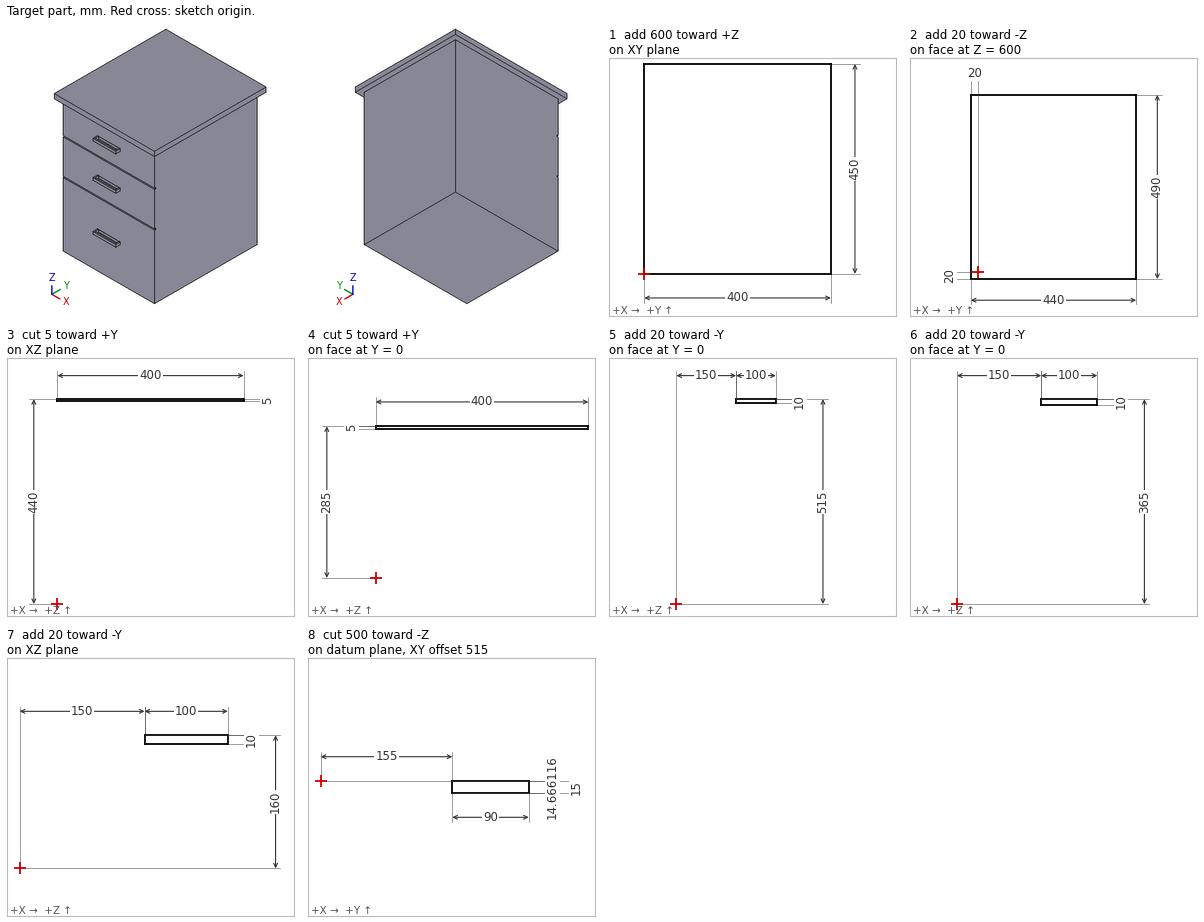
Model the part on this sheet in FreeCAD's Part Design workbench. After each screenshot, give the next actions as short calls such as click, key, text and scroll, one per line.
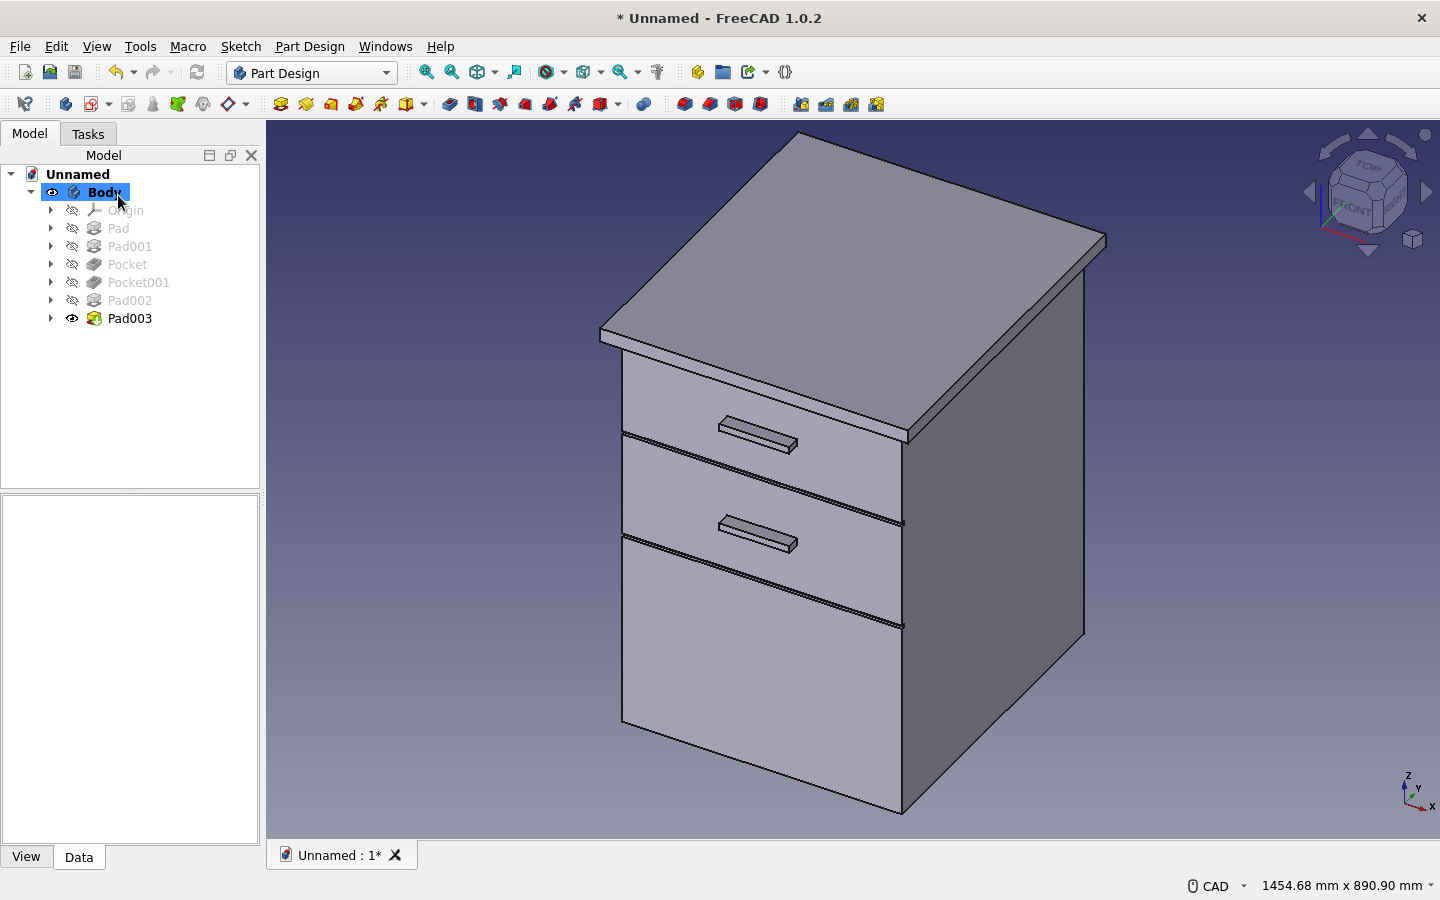
click(90, 104)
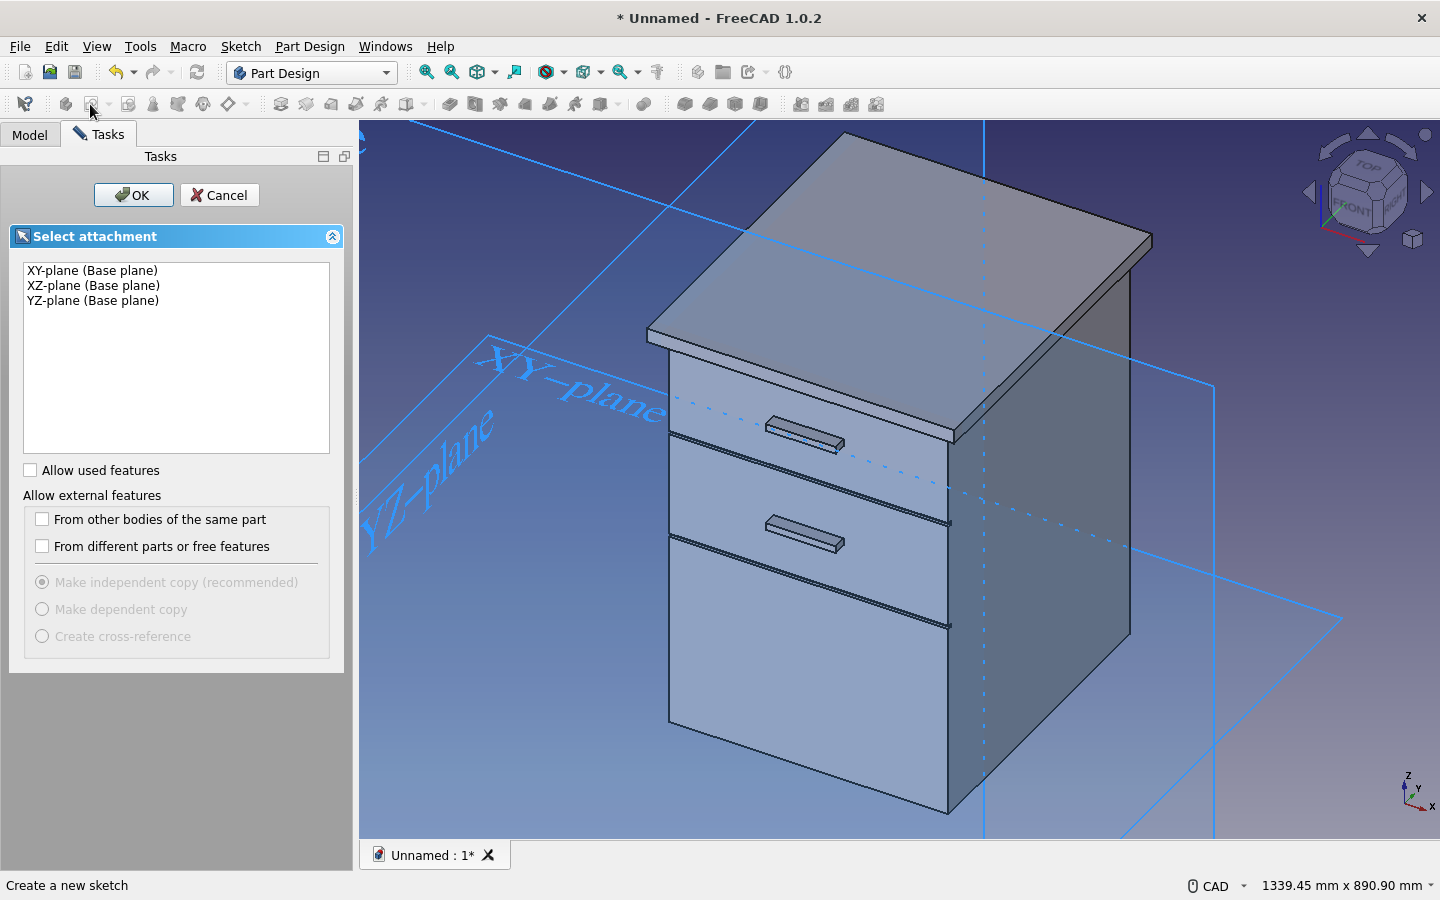
click(84, 286)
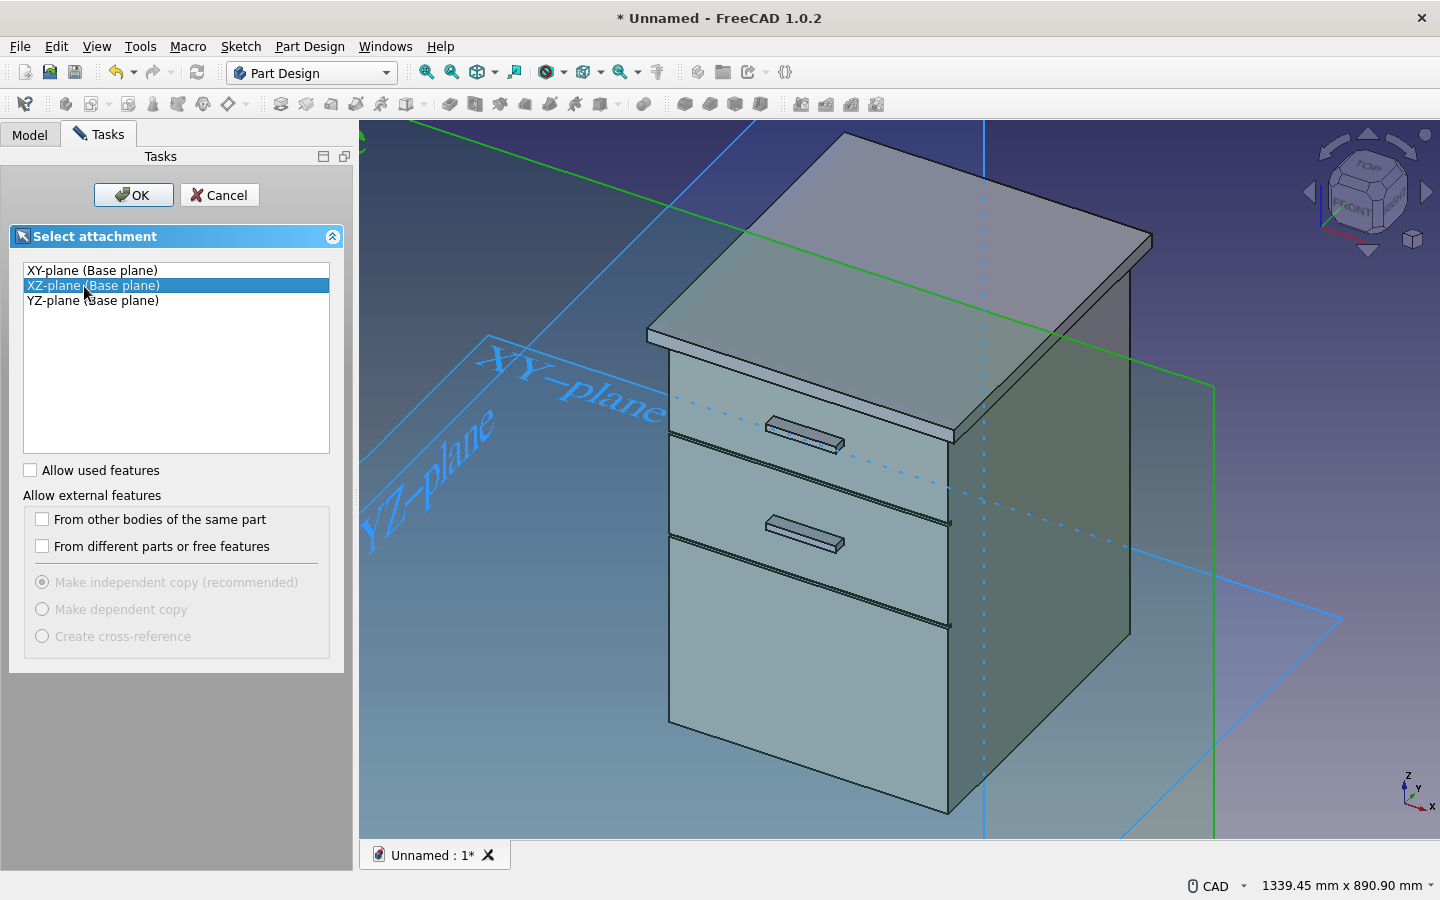
click(134, 195)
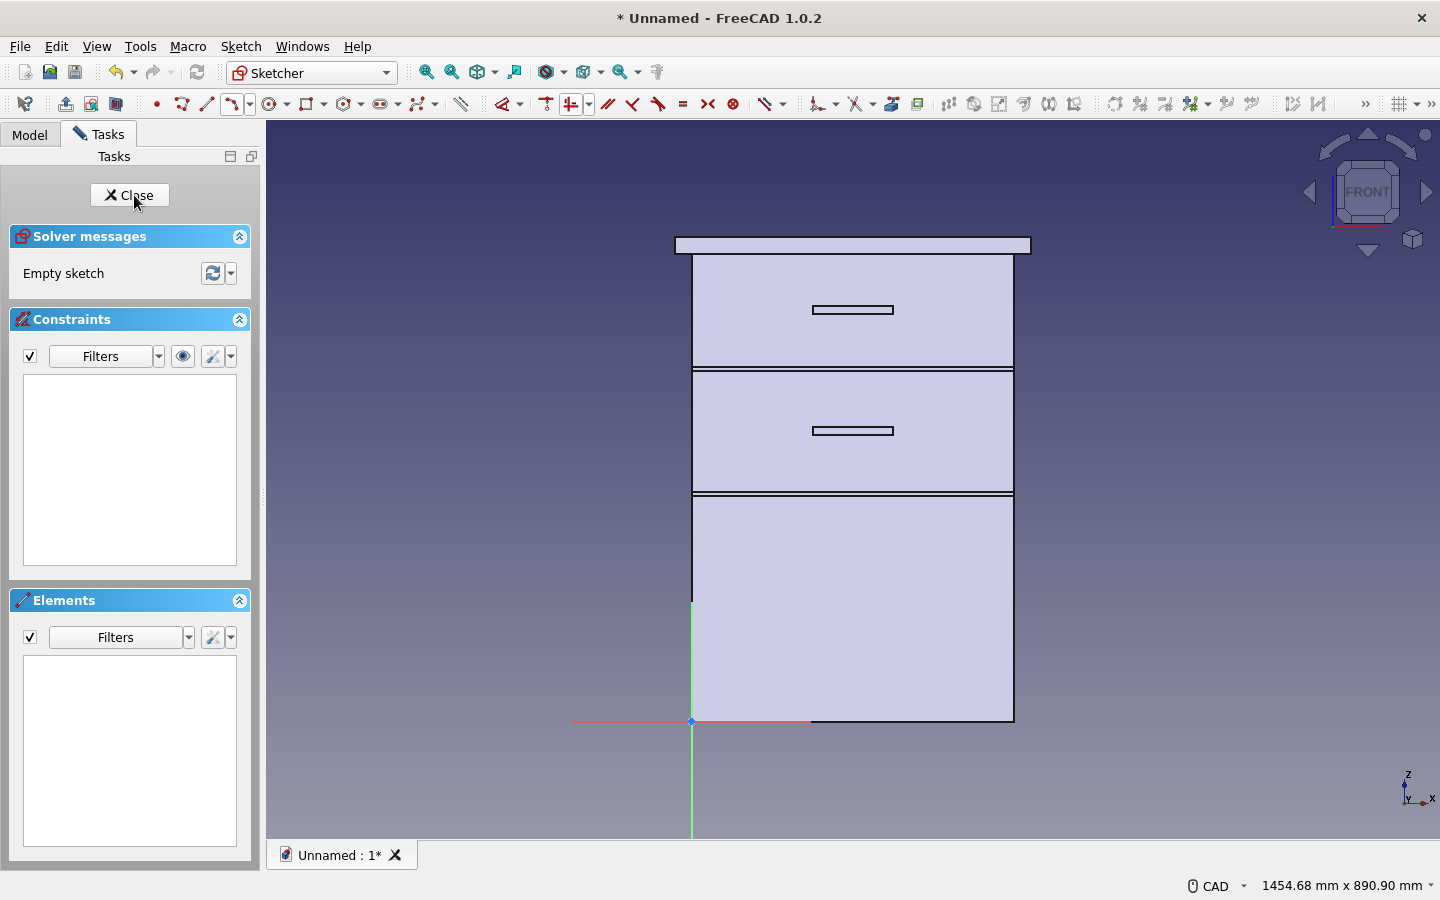
click(116, 104)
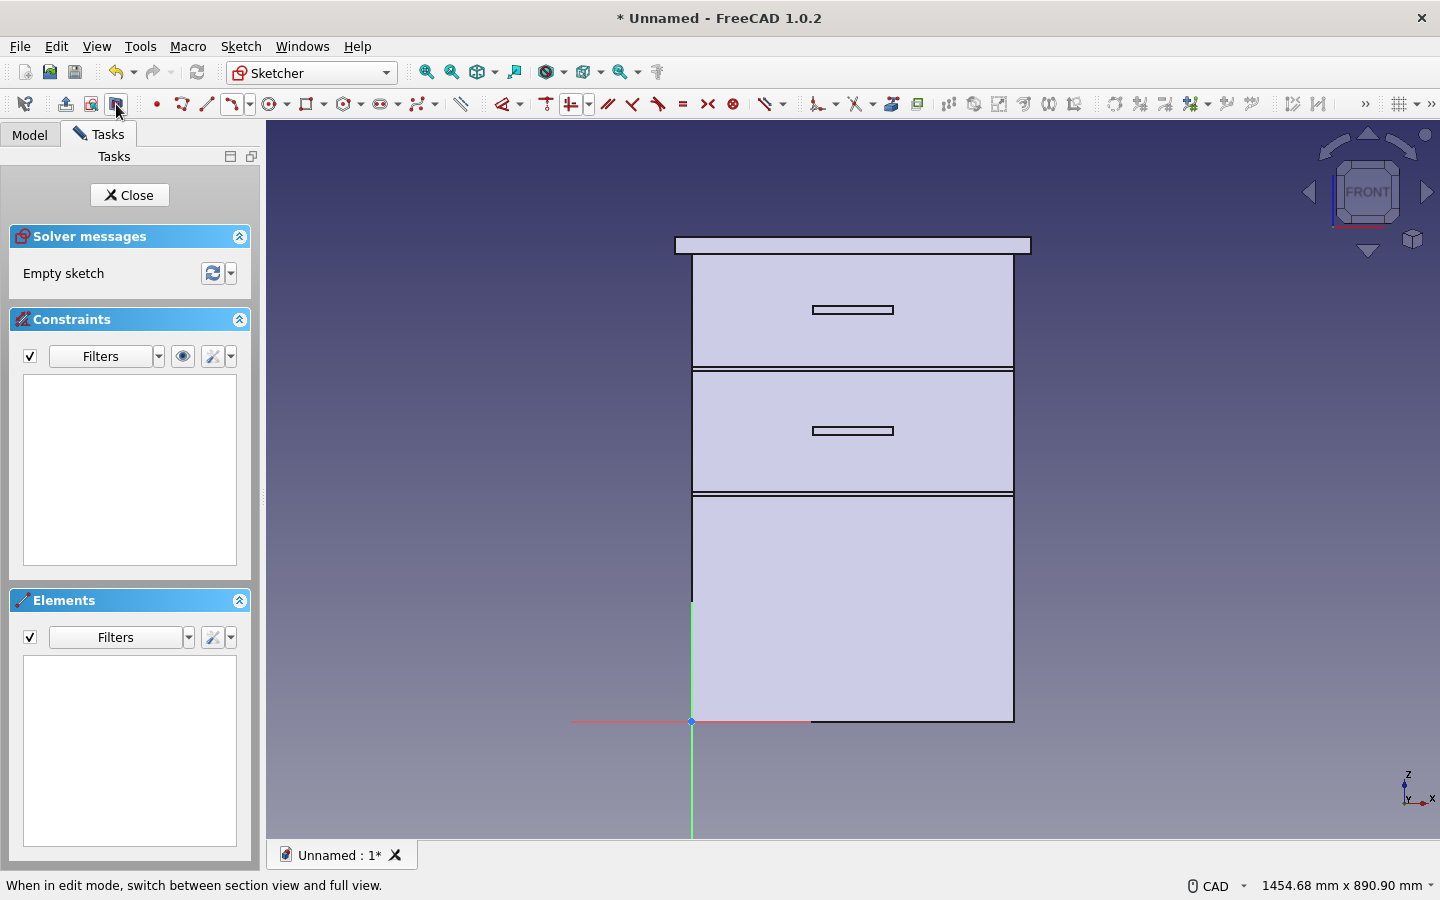
scroll(862, 611, up, 11)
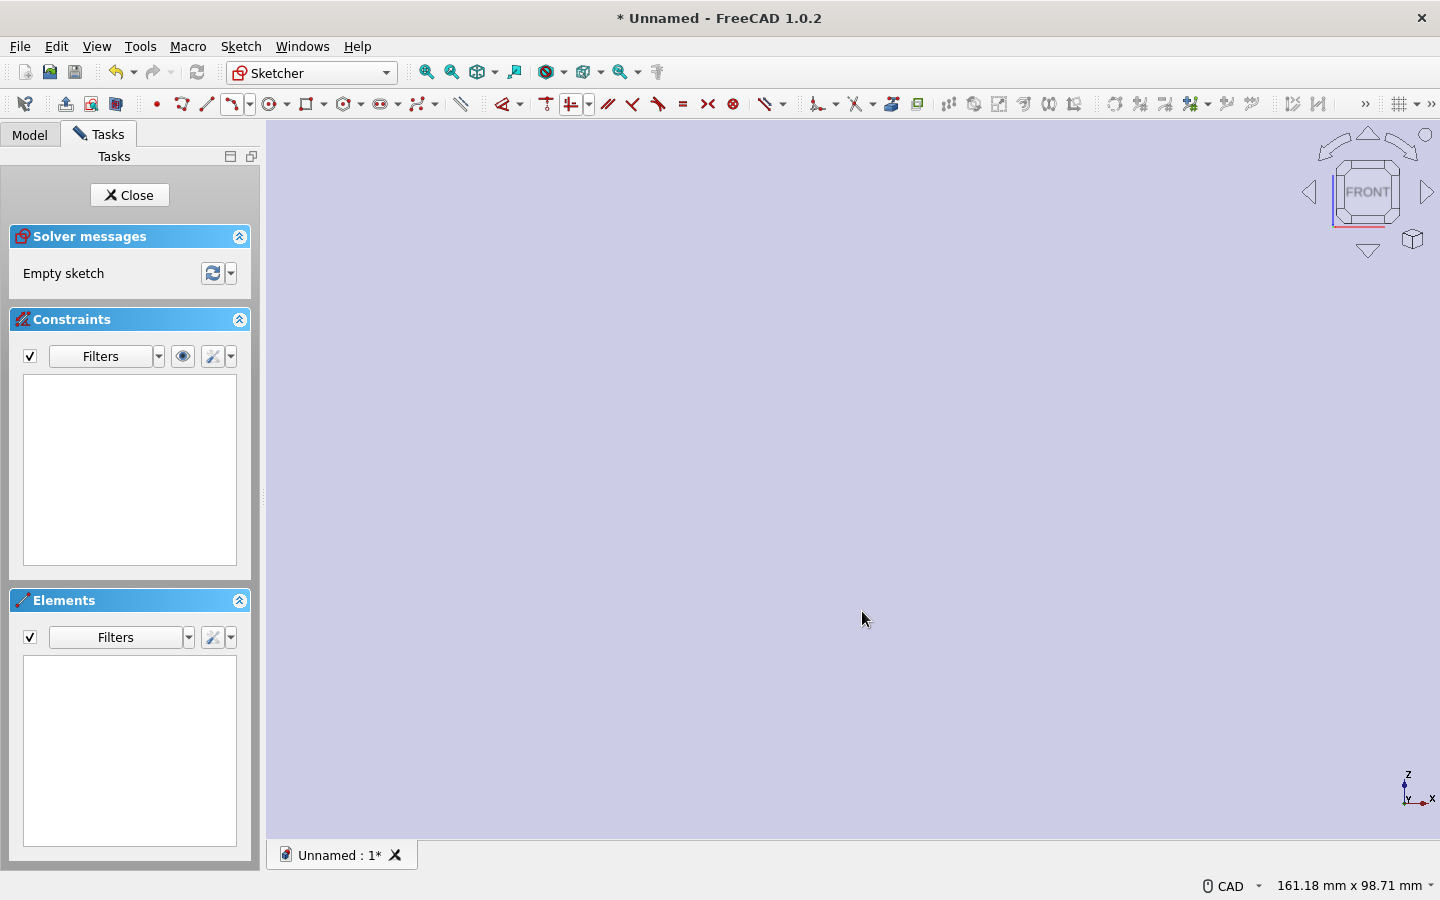
click(306, 104)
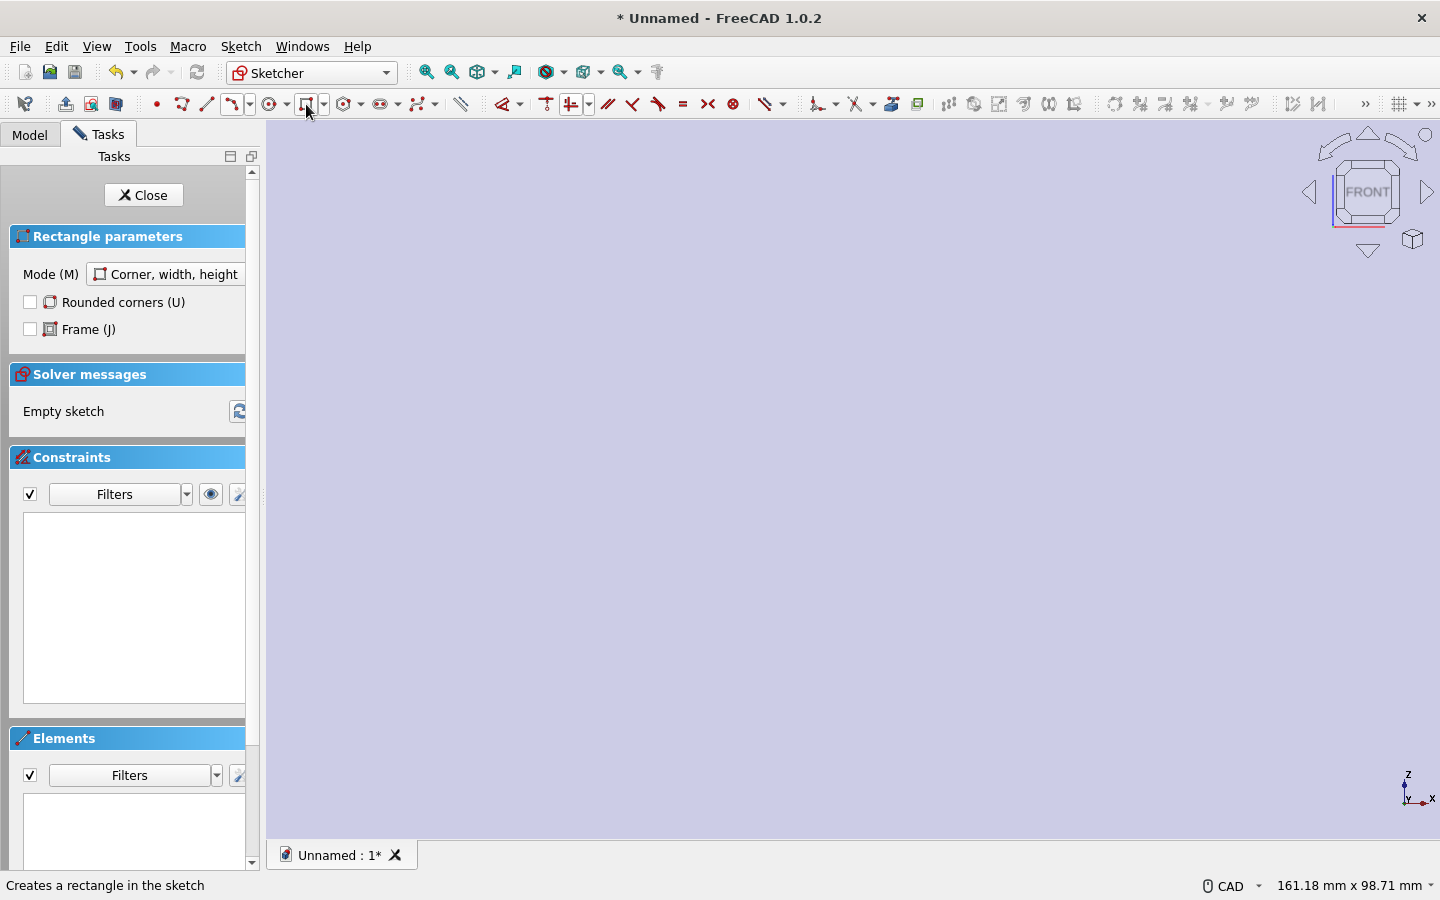
click(413, 438)
move(1141, 511)